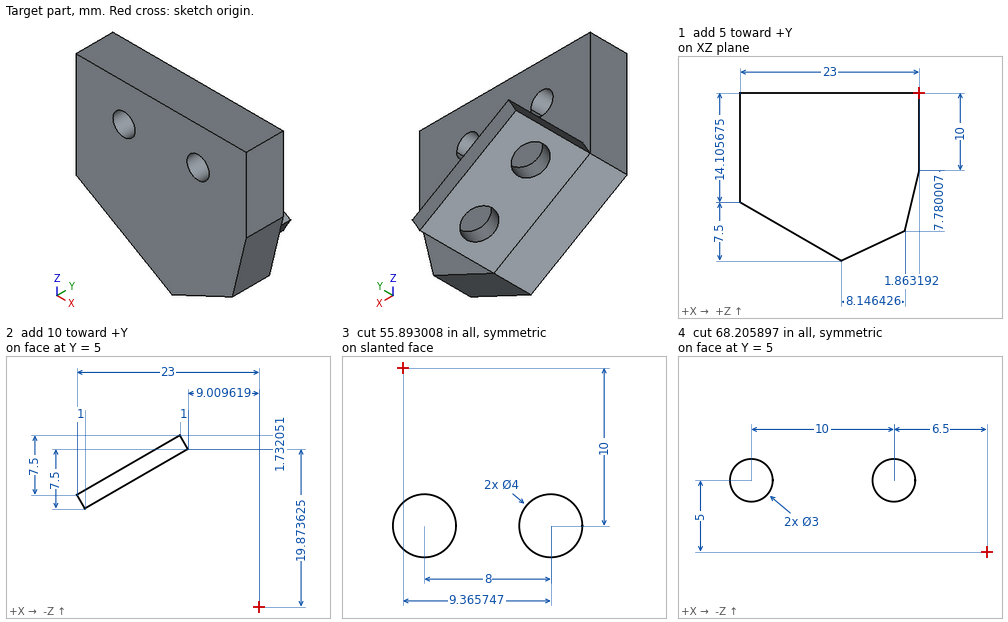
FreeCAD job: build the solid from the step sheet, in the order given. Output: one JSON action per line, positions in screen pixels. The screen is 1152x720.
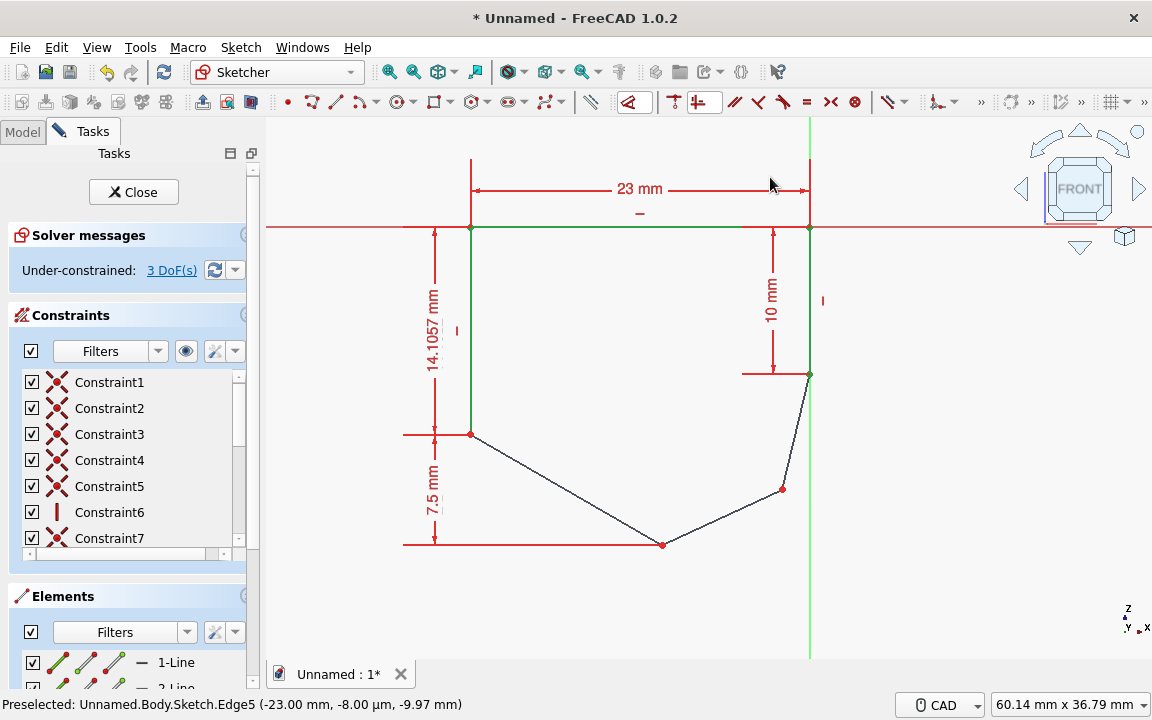
{"action": "scroll", "coordinate": [782, 490], "scroll_direction": "up", "scroll_amount": 2}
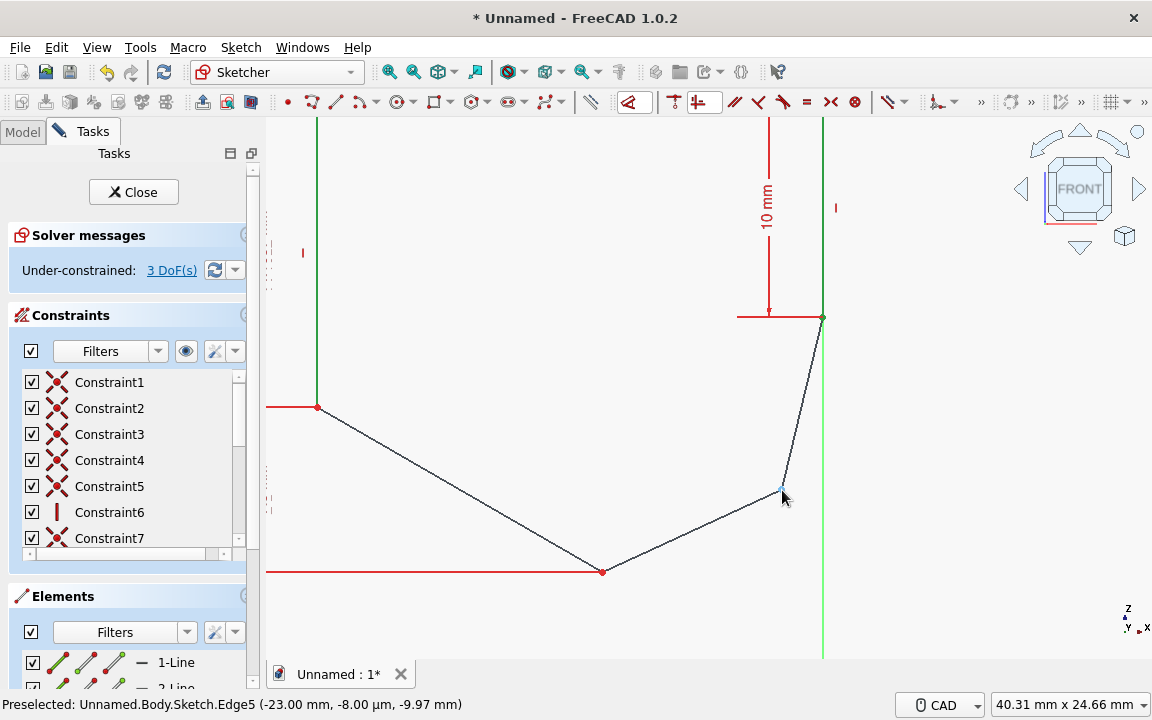
{"action": "left_click", "coordinate": [782, 490]}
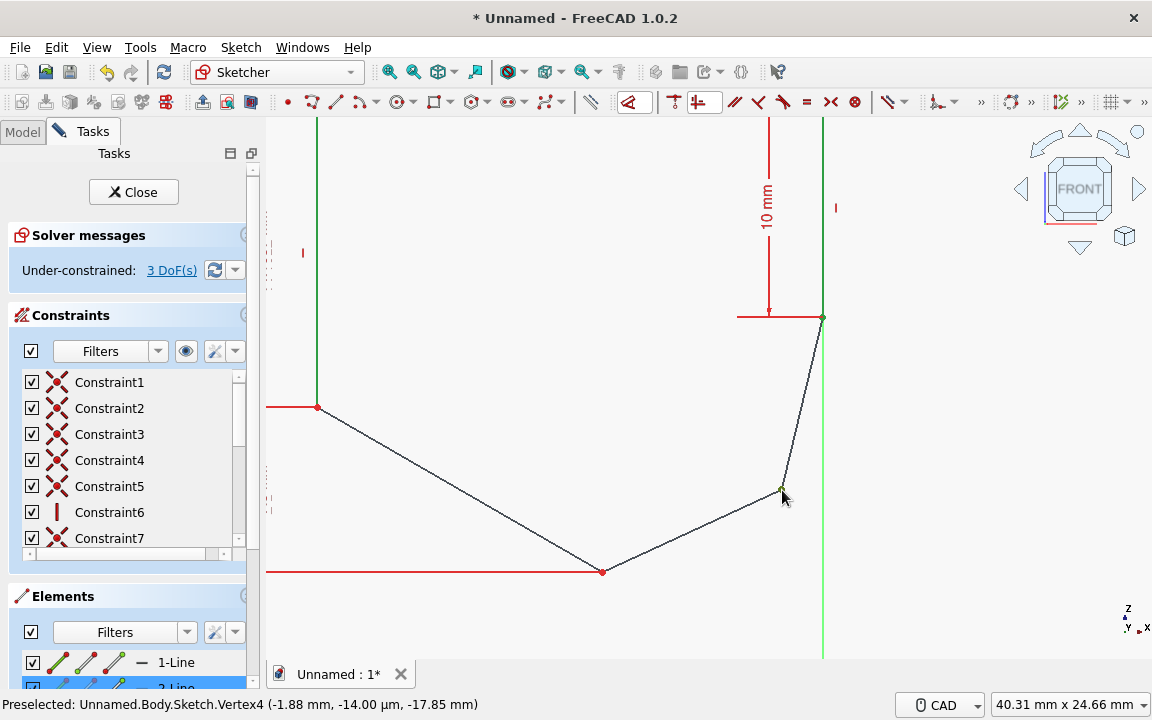
{"action": "left_click", "coordinate": [646, 102]}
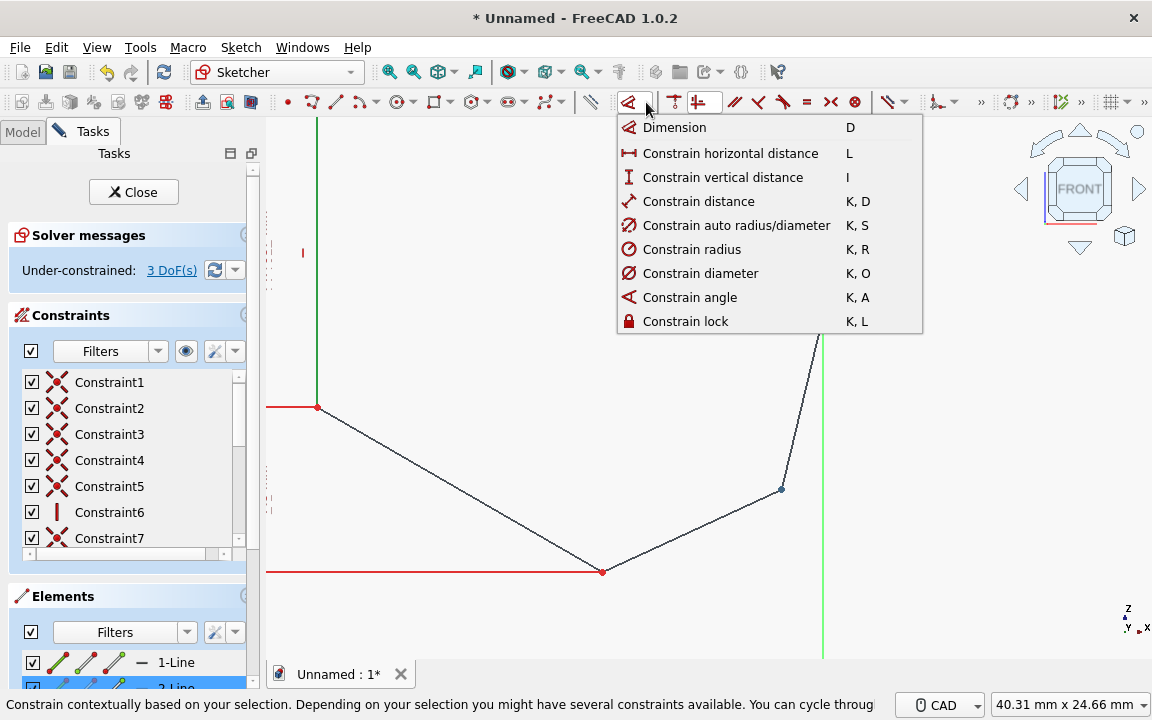
{"action": "left_click", "coordinate": [770, 153]}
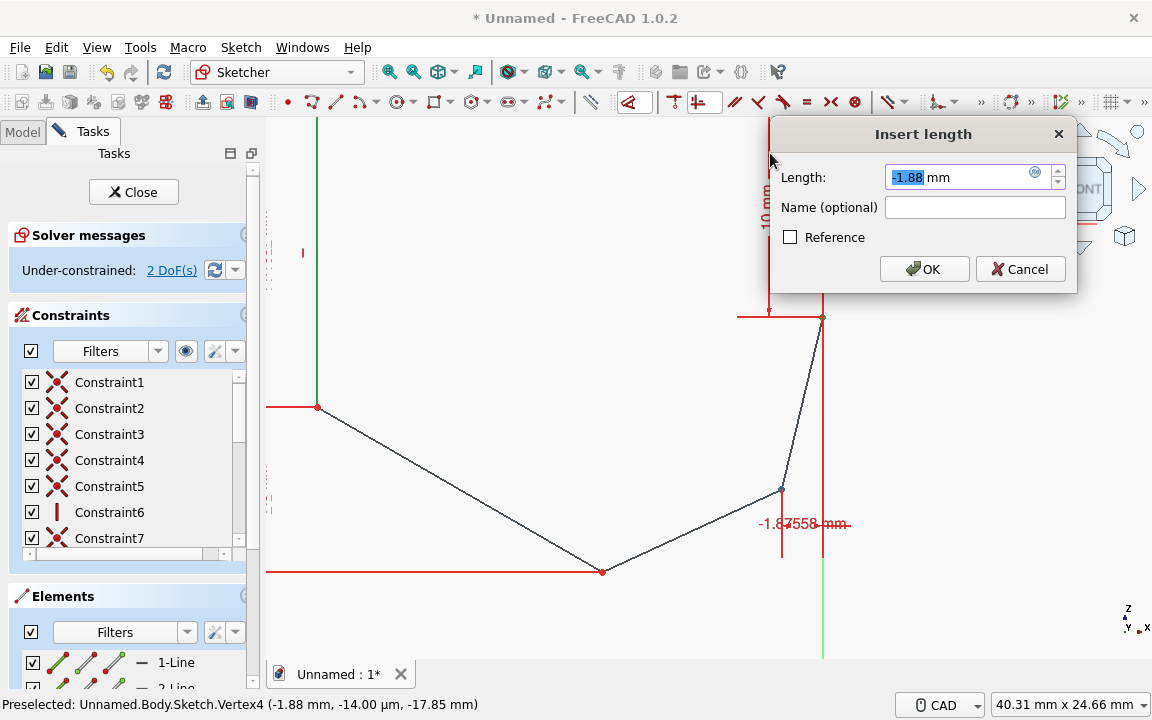
{"action": "type", "text": "-1.863192"}
{"action": "key", "text": "Return"}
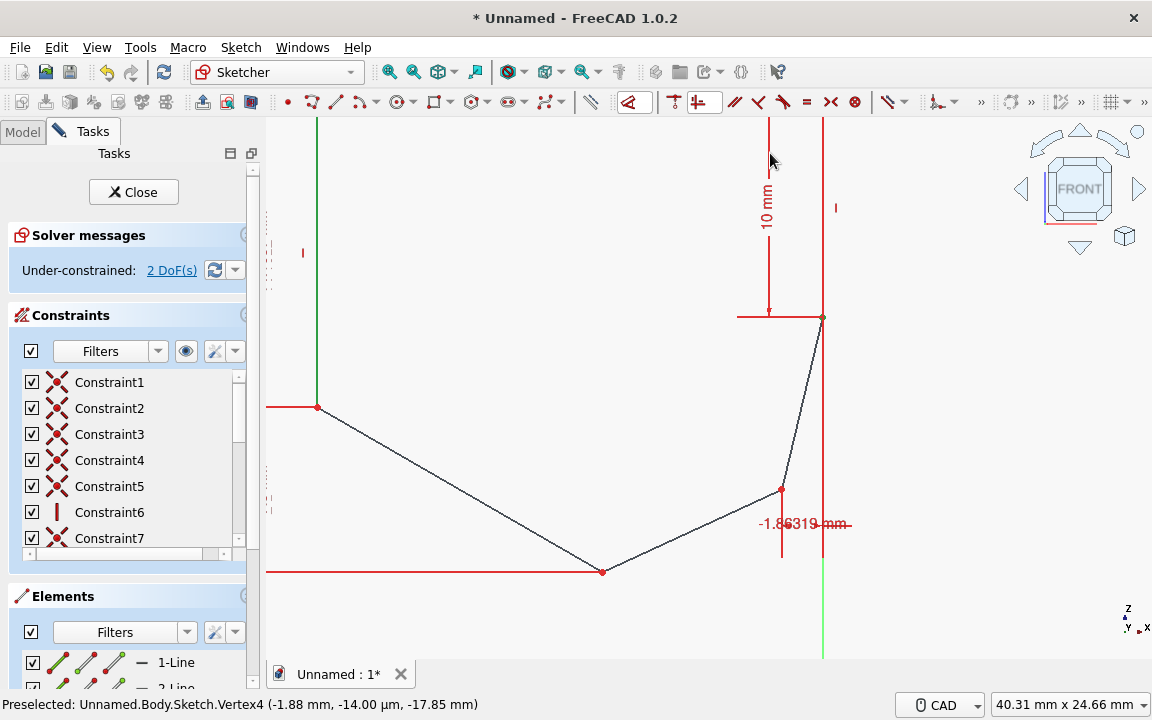
{"action": "left_click", "coordinate": [811, 369]}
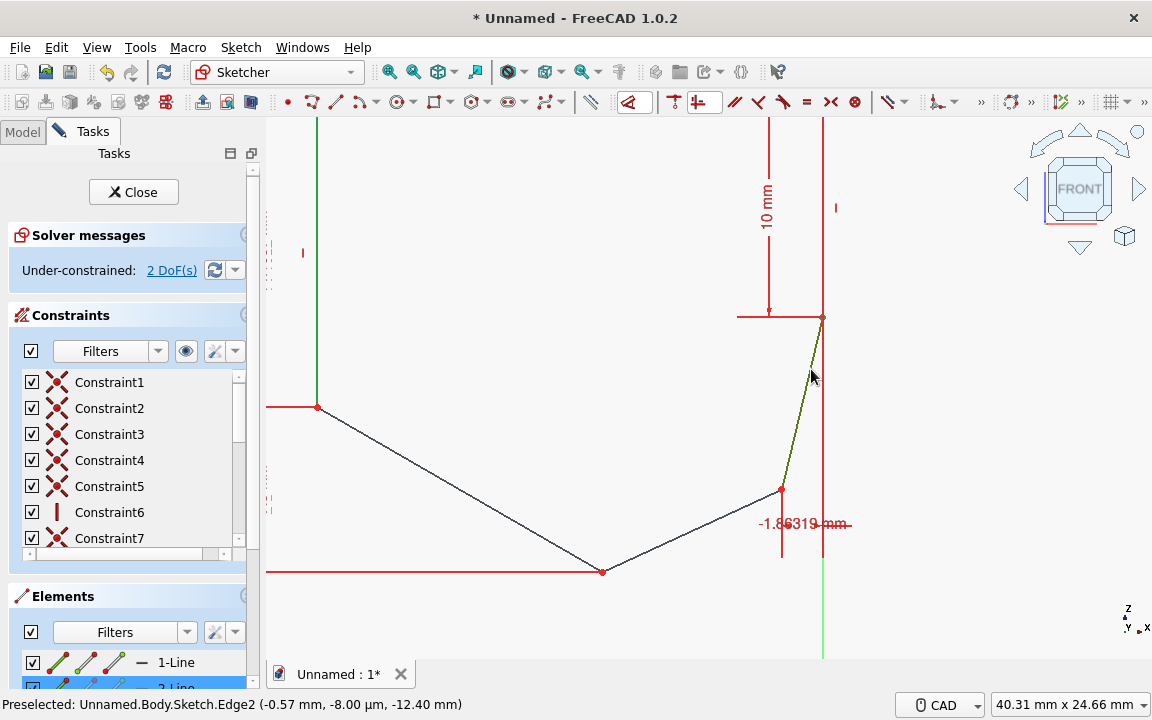
{"action": "left_click", "coordinate": [646, 102]}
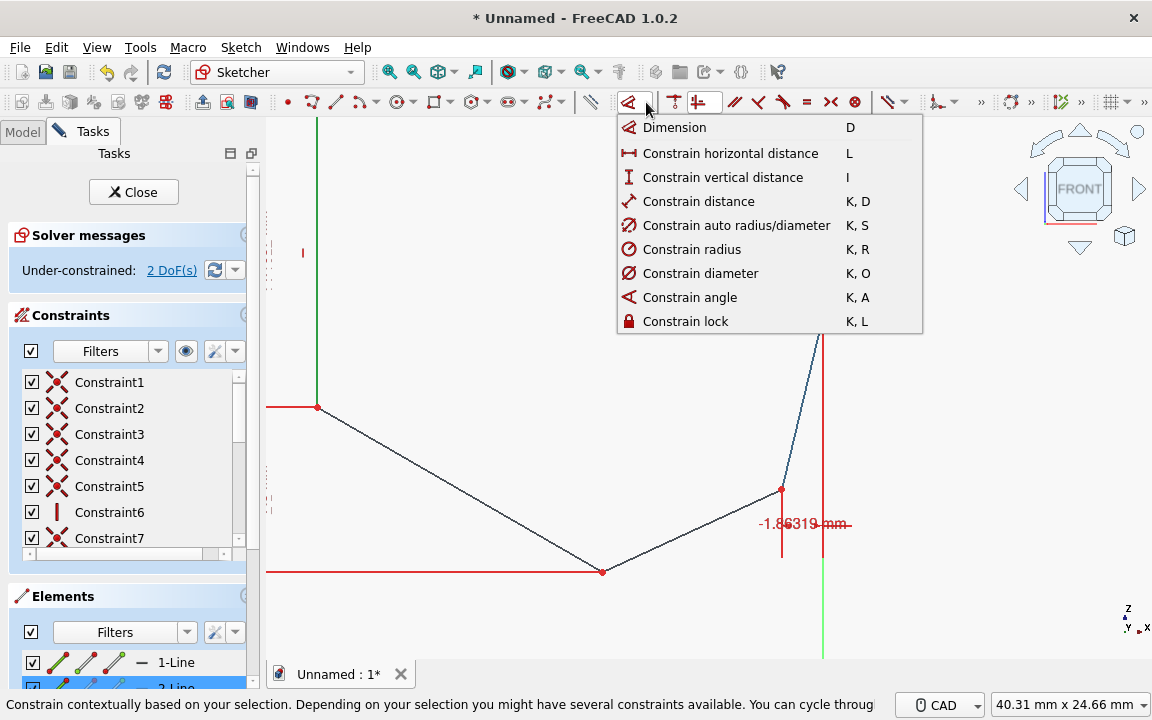
{"action": "left_click", "coordinate": [770, 177]}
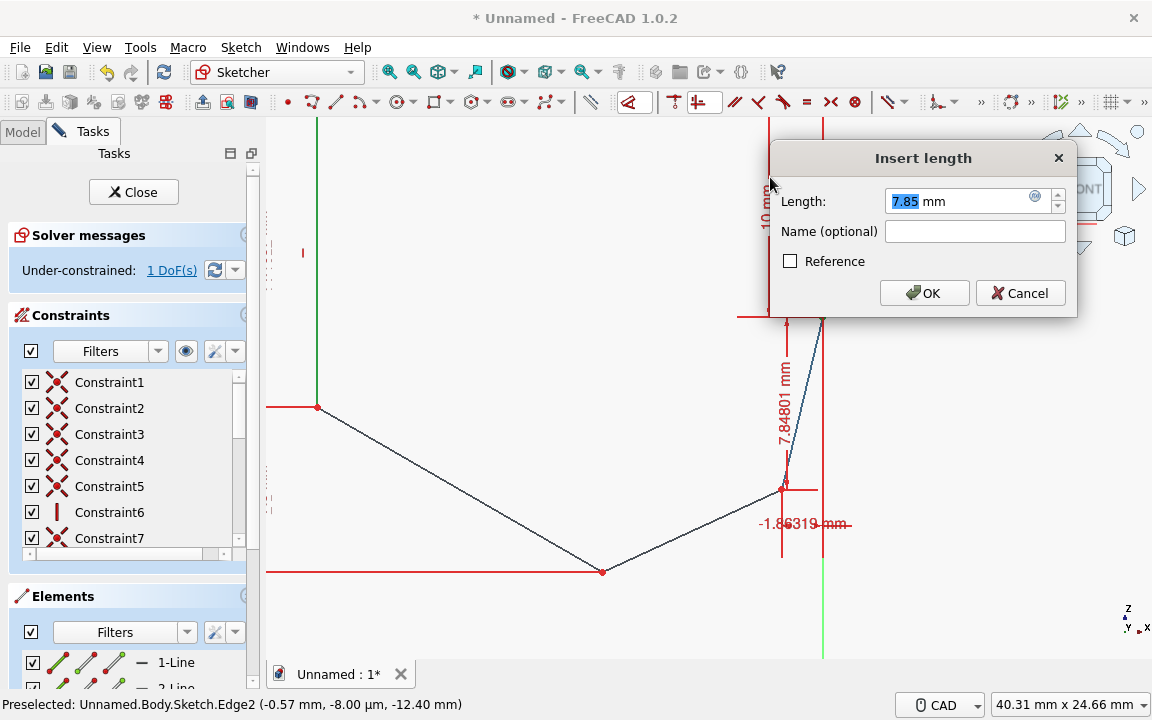
{"action": "type", "text": "7.780007"}
{"action": "key", "text": "Return"}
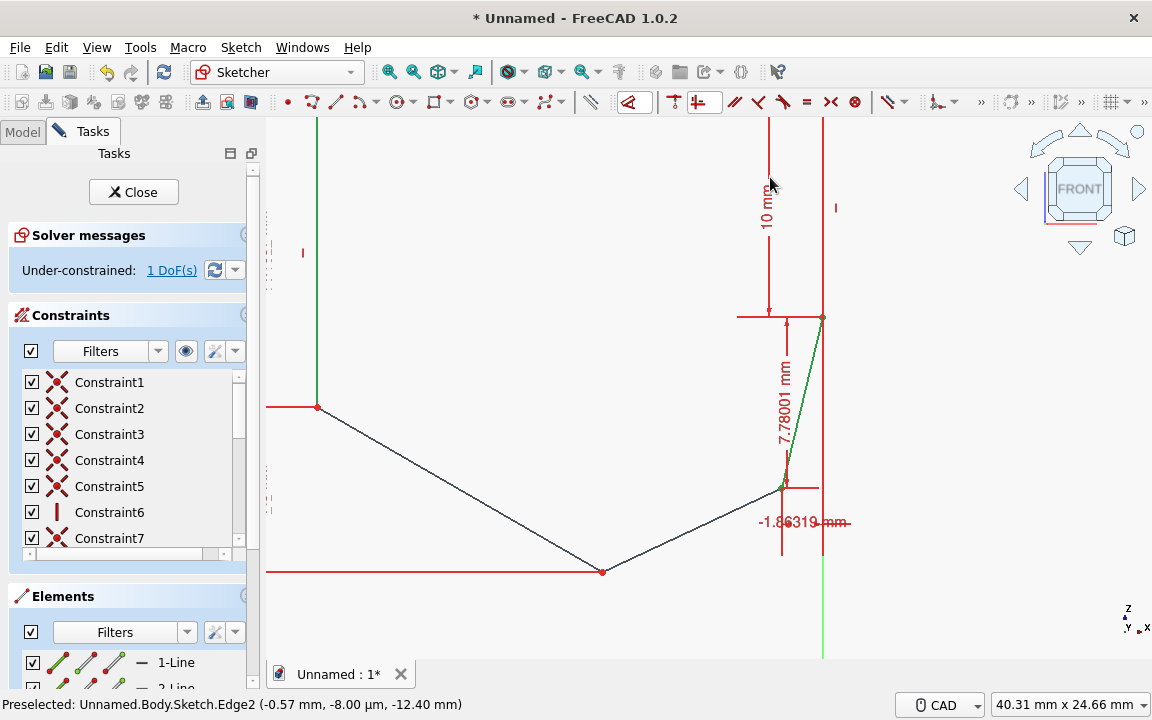
{"action": "left_click", "coordinate": [728, 513]}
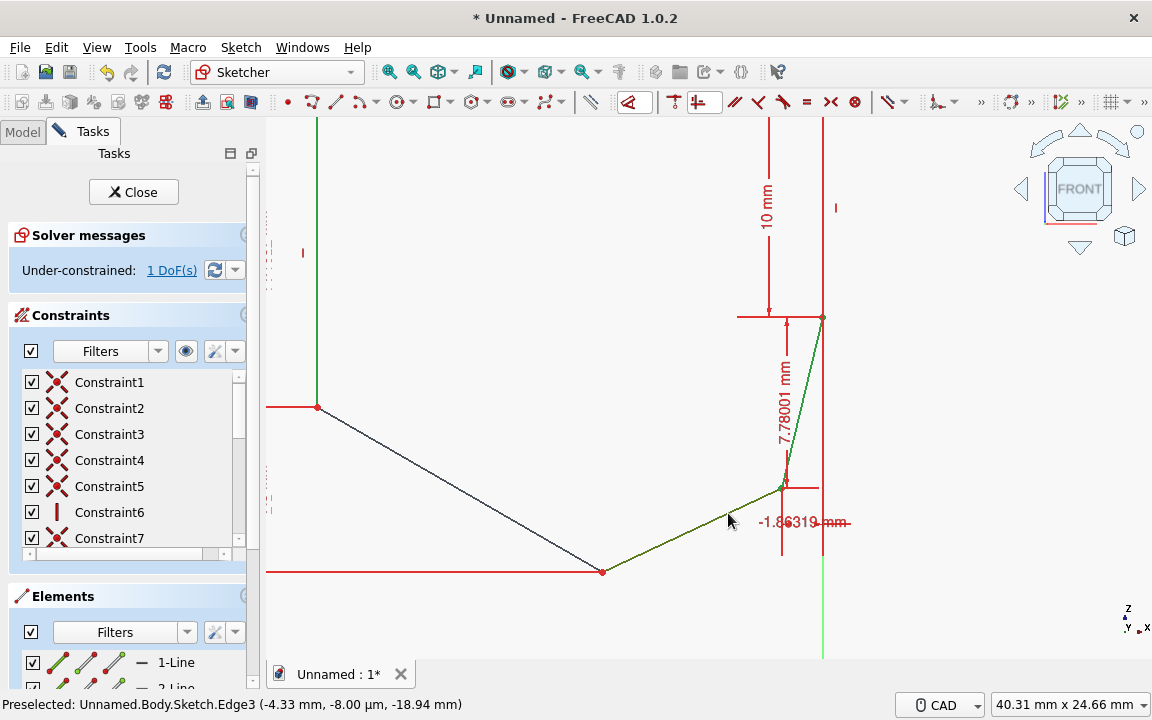
{"action": "left_click", "coordinate": [646, 102]}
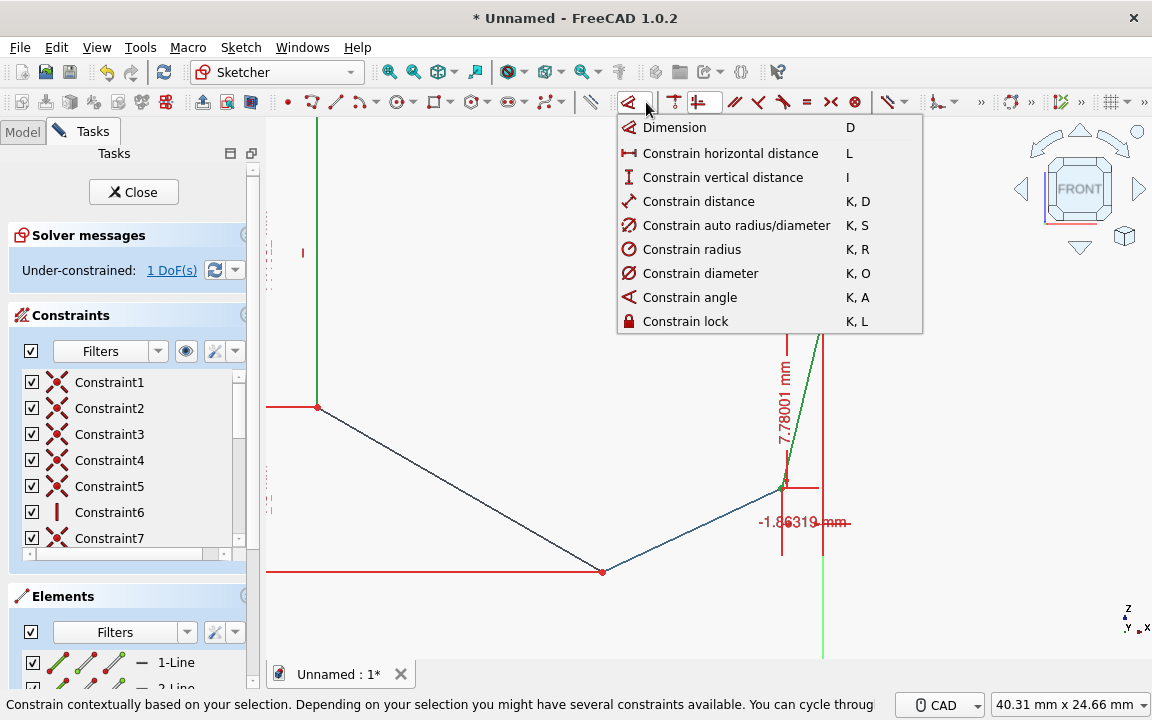
{"action": "left_click", "coordinate": [770, 153]}